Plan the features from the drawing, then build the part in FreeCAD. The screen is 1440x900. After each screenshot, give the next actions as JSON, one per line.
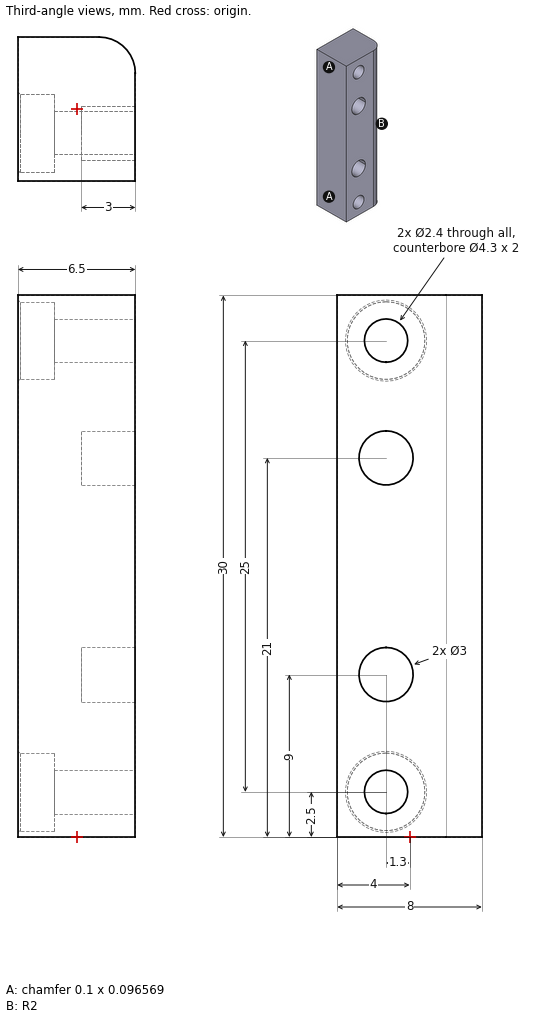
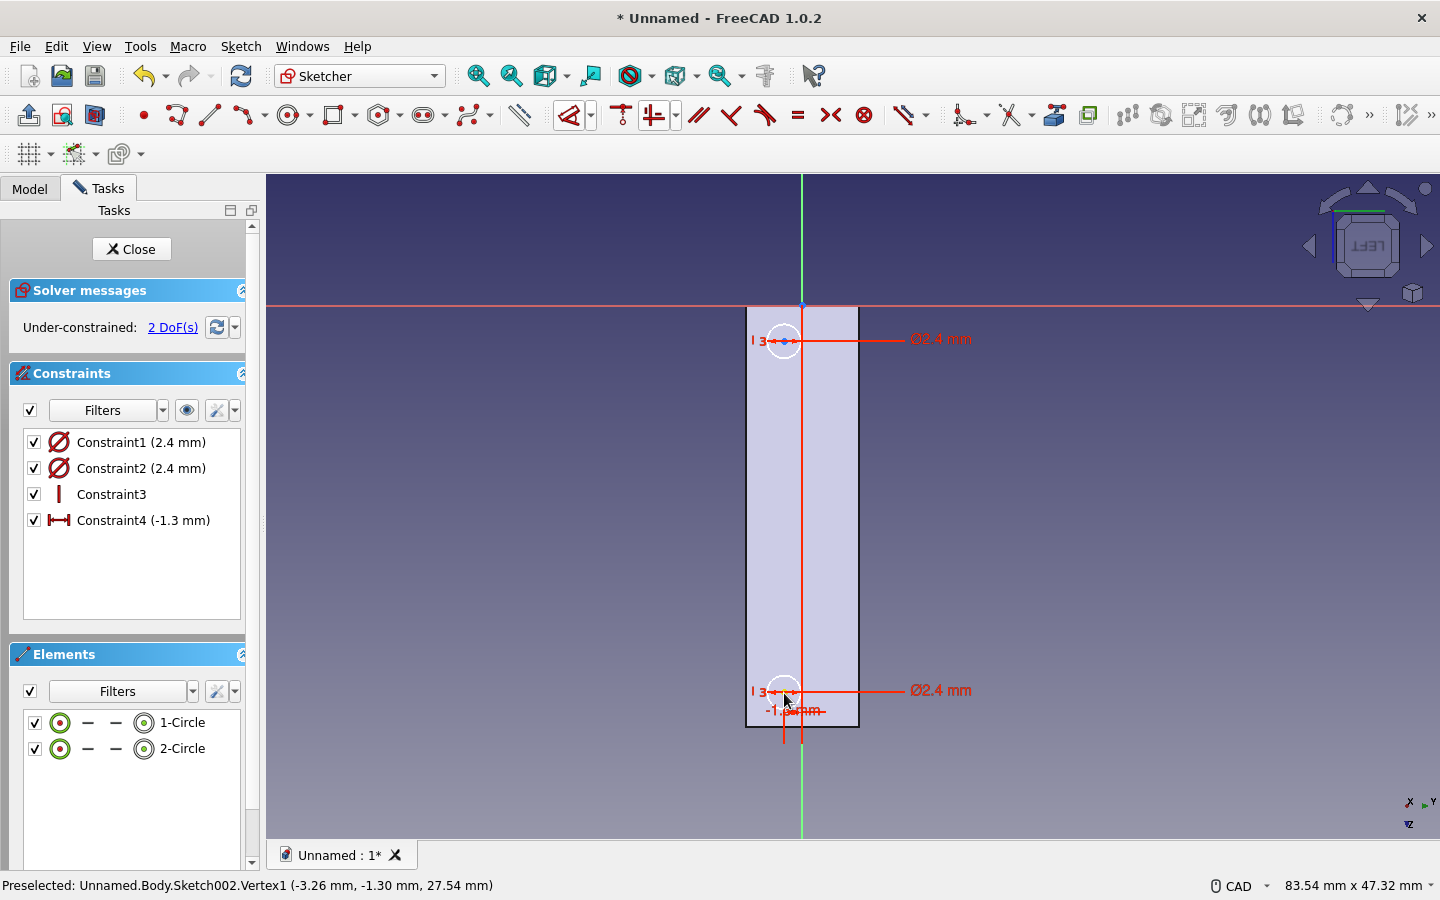
{"action": "left_click", "coordinate": [784, 341]}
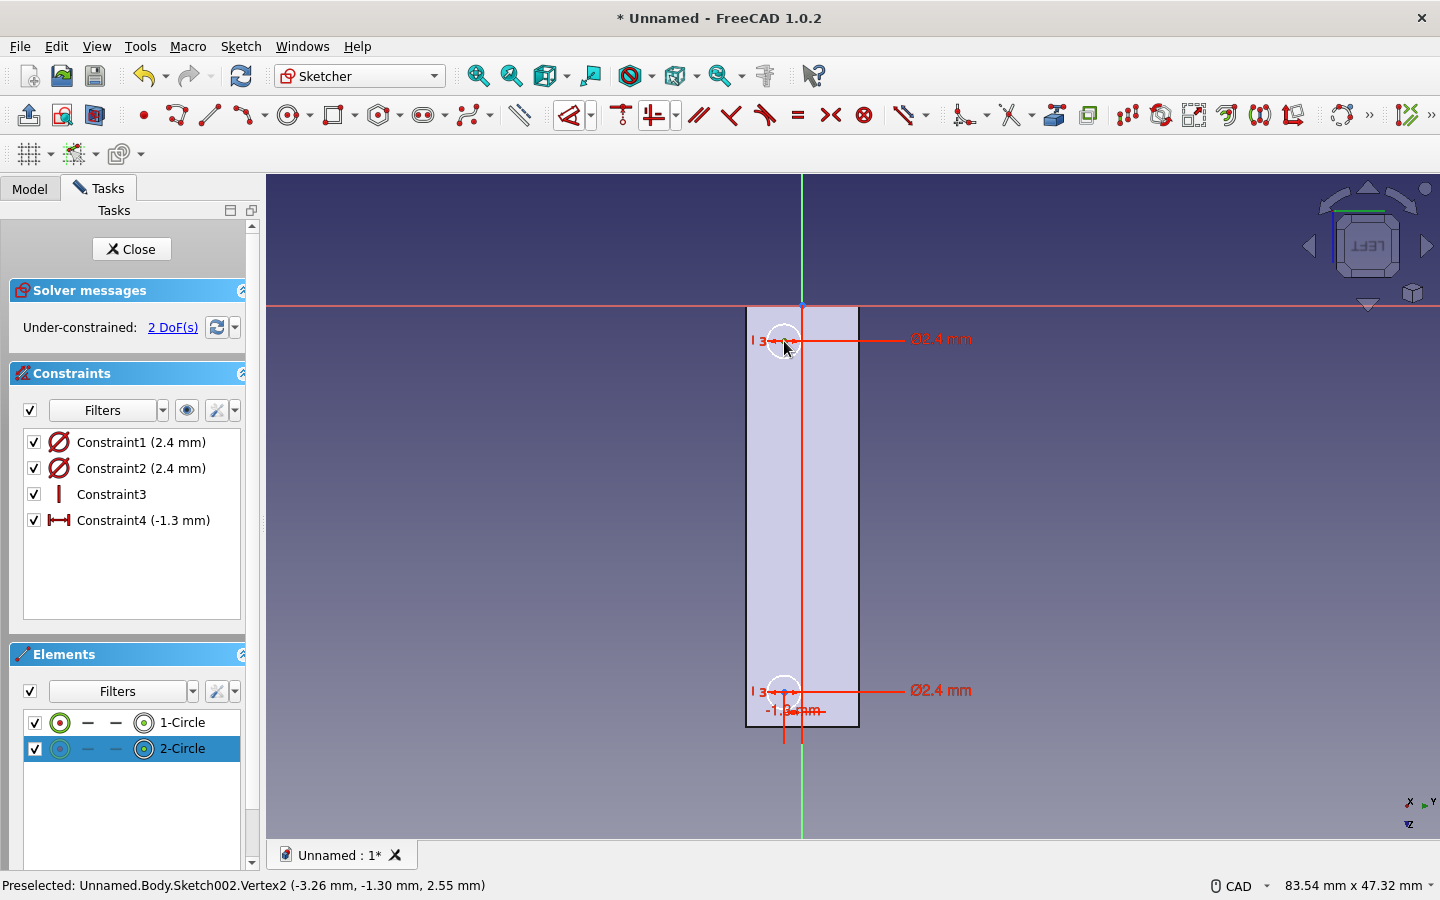
{"action": "left_click", "coordinate": [590, 116]}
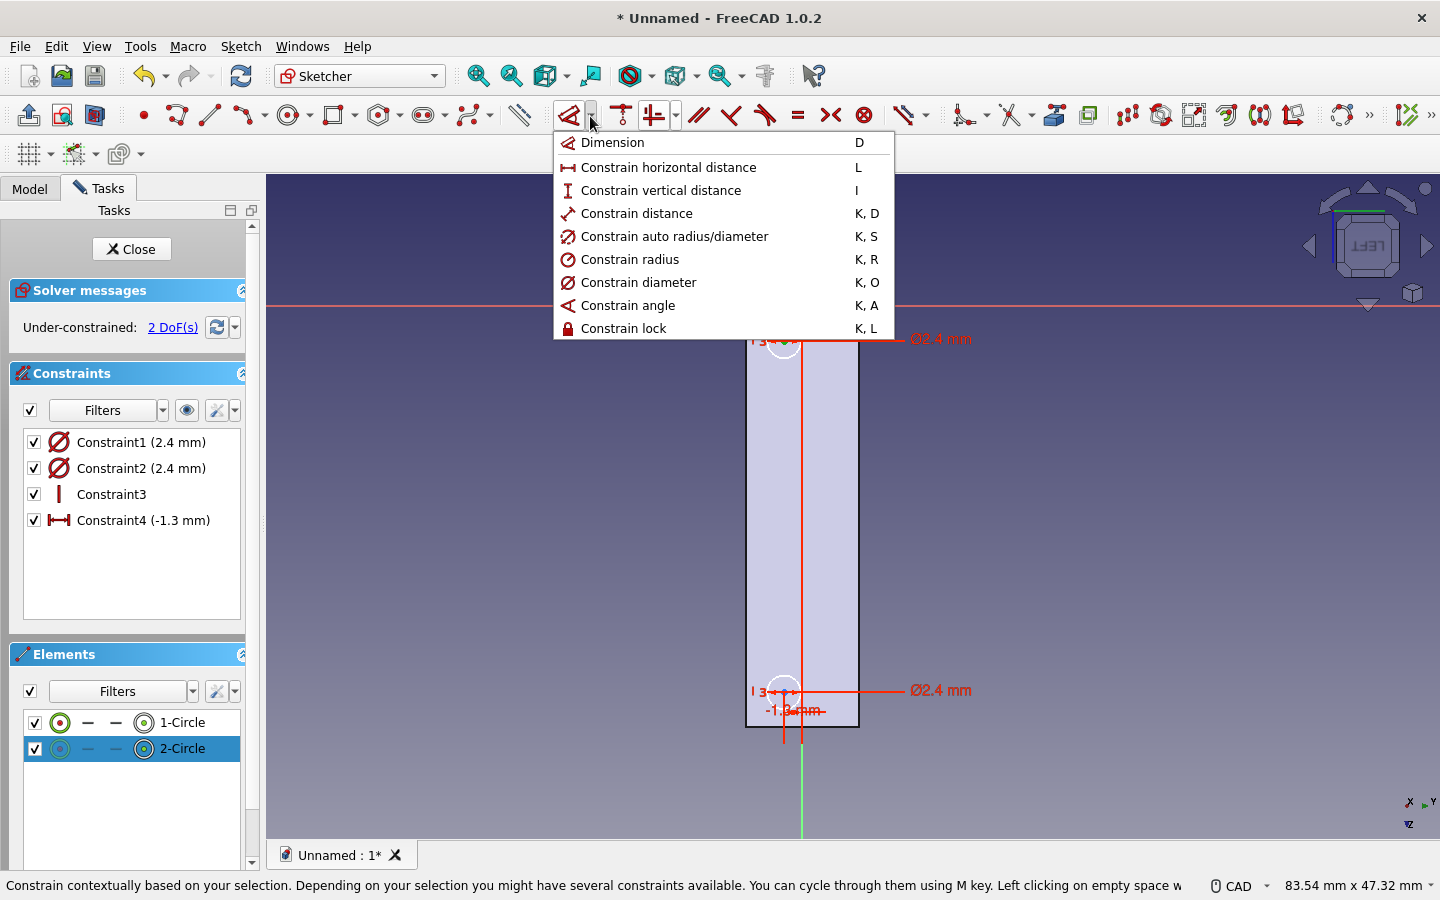
{"action": "left_click", "coordinate": [724, 190]}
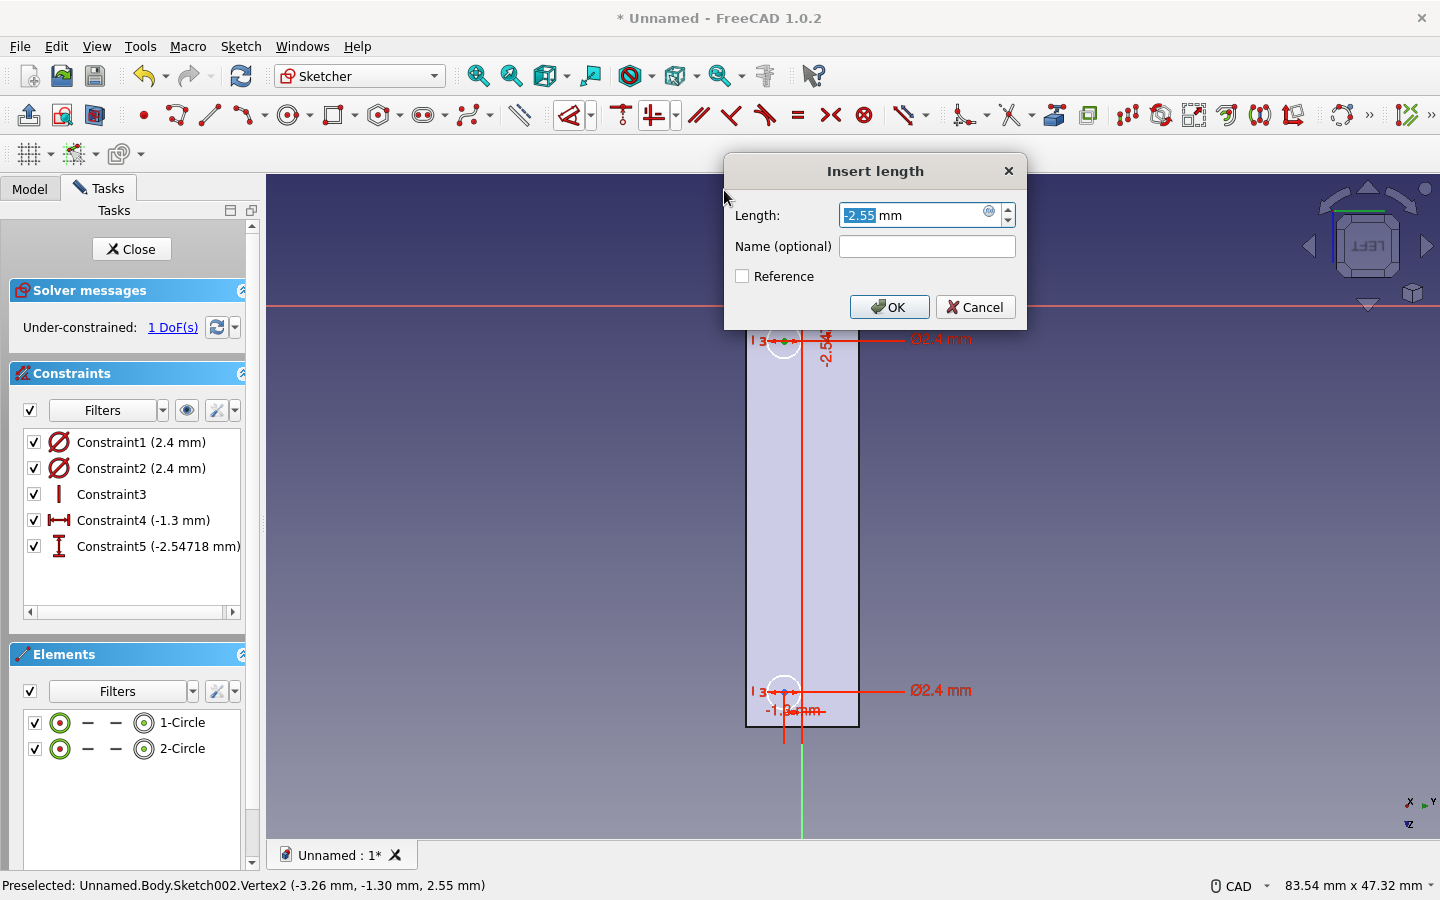
{"action": "type", "text": "-2.5"}
{"action": "key", "text": "Return"}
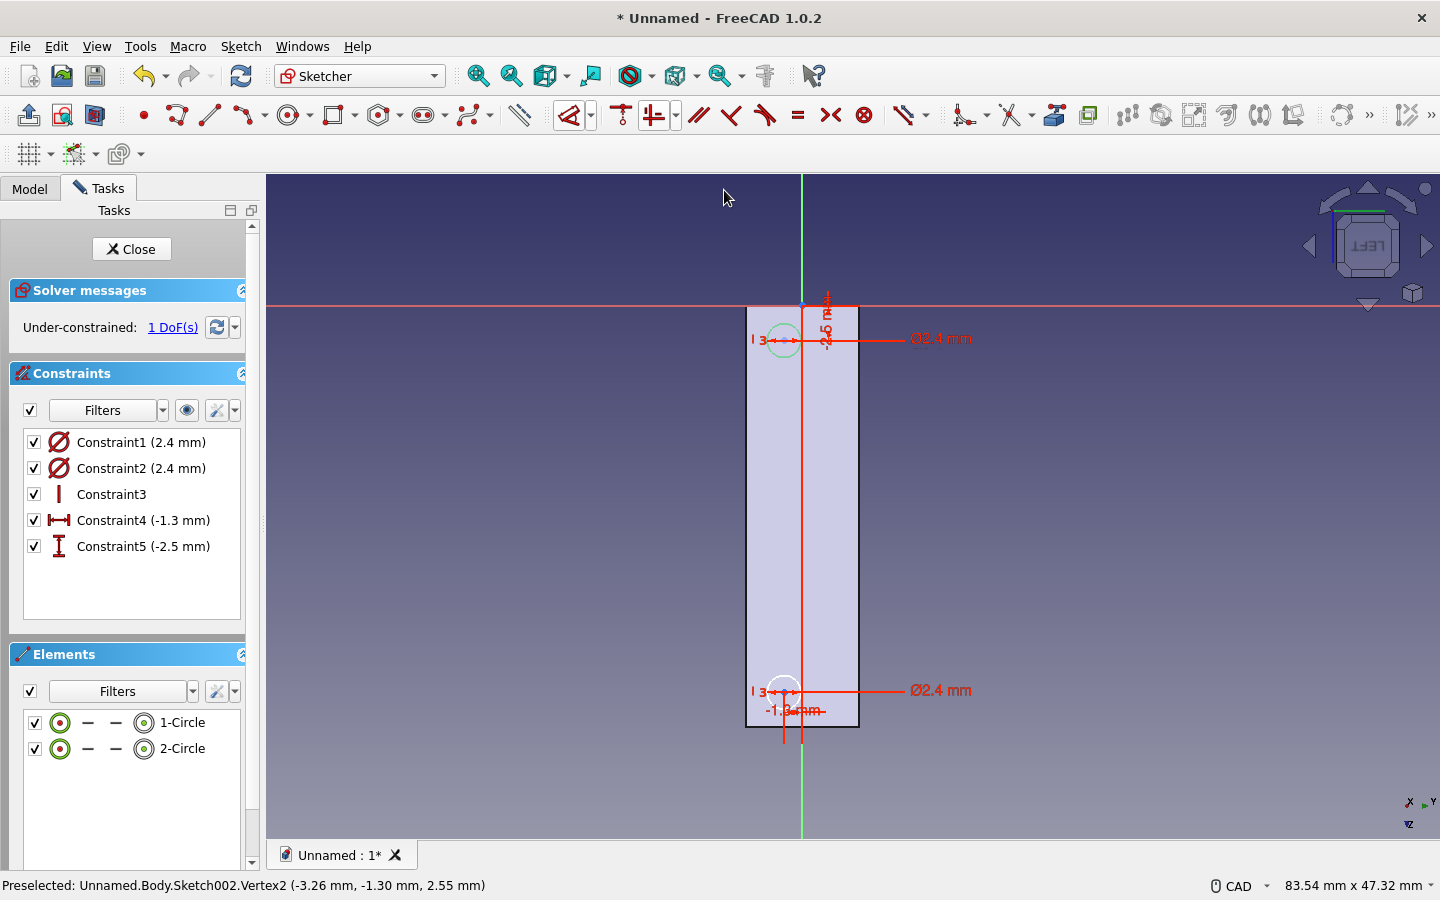
{"action": "left_click", "coordinate": [784, 692]}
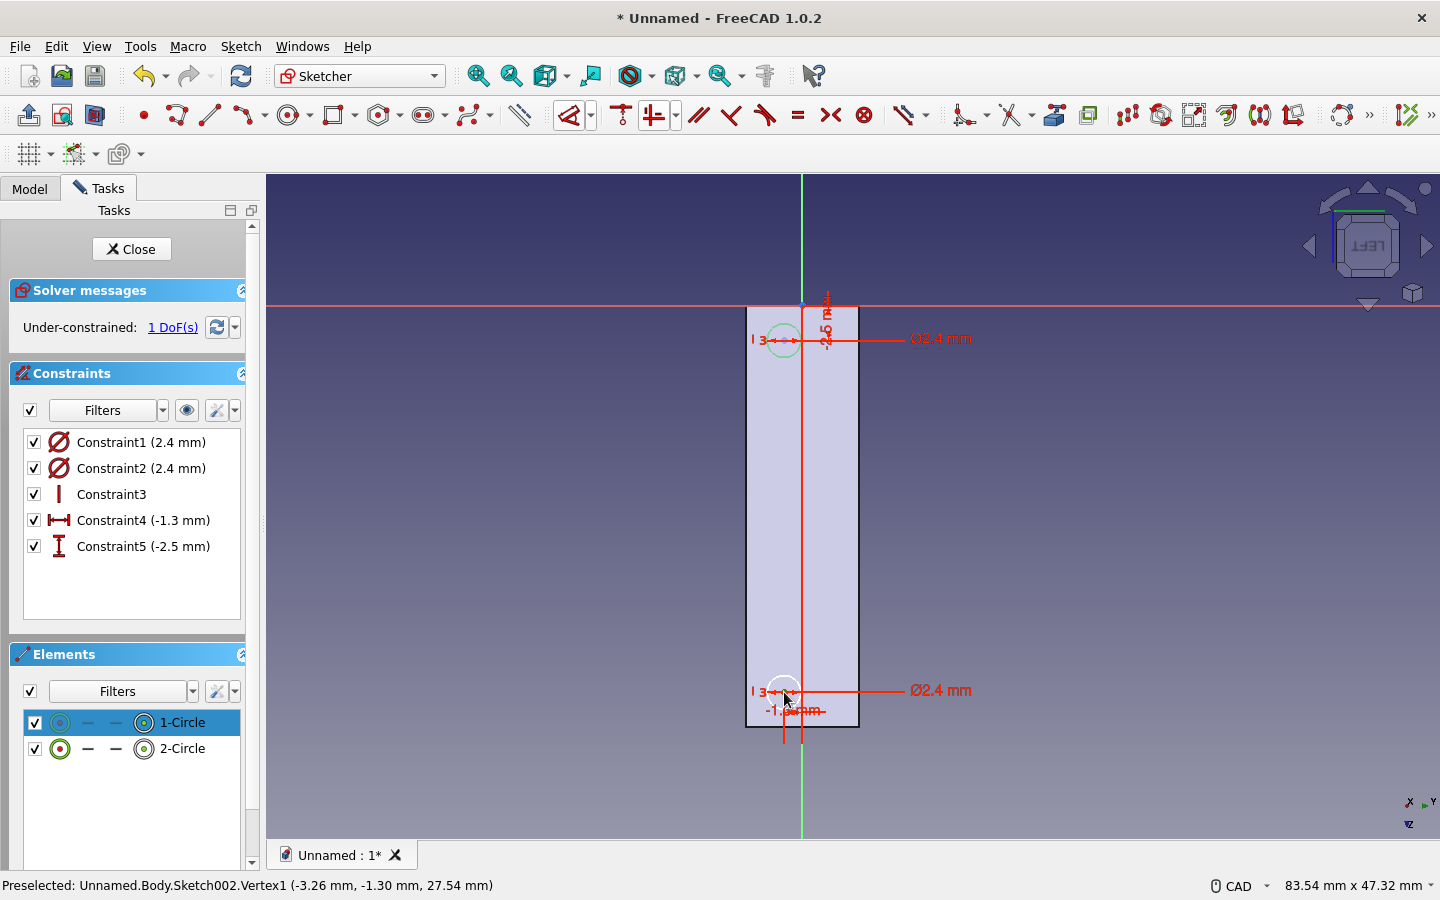
{"action": "left_click", "coordinate": [784, 341]}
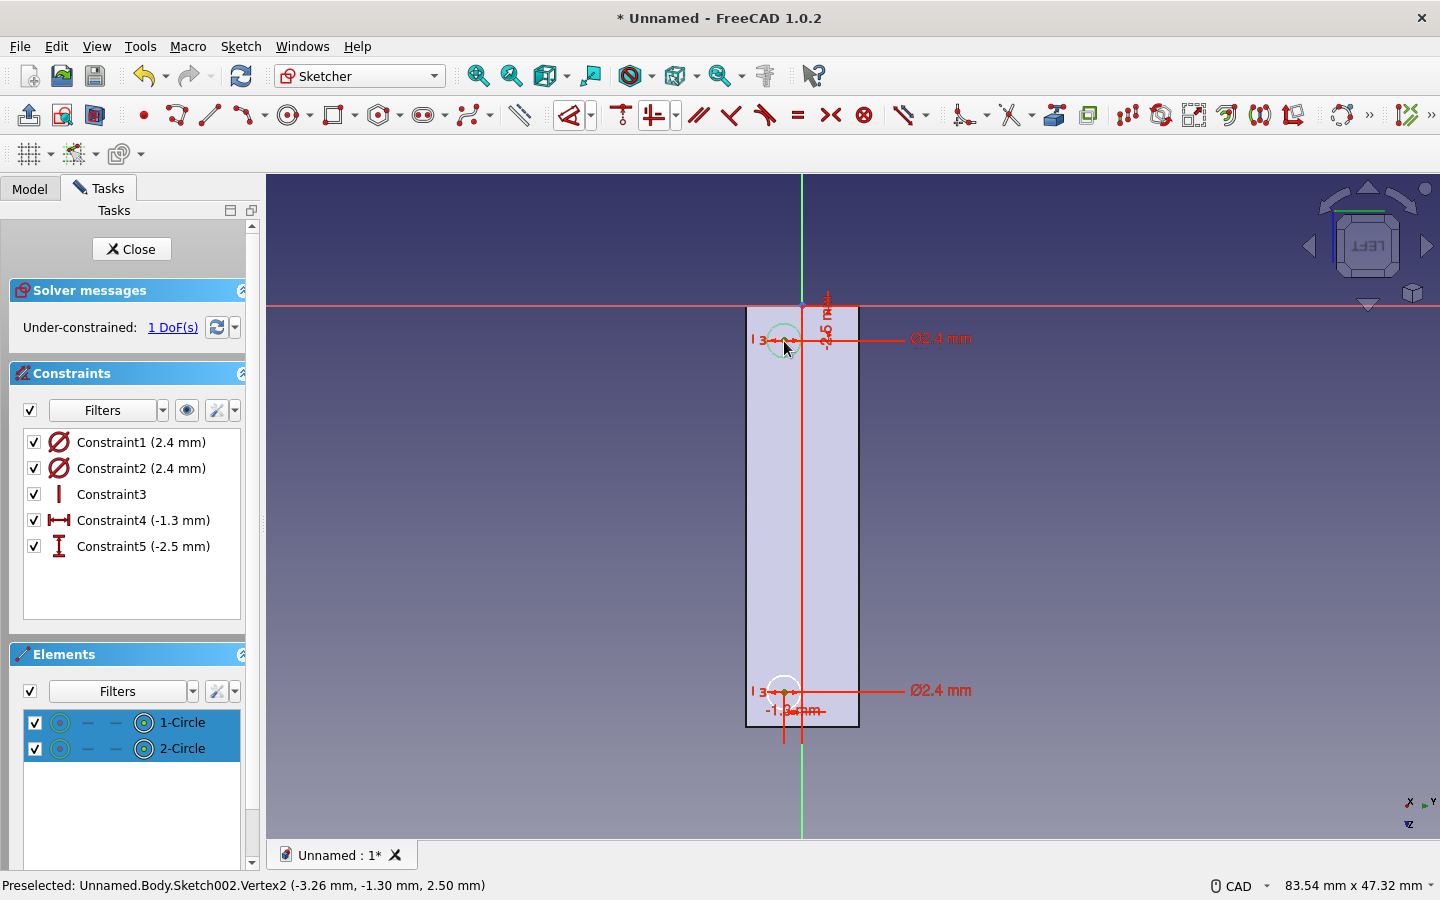
{"action": "left_click", "coordinate": [590, 116]}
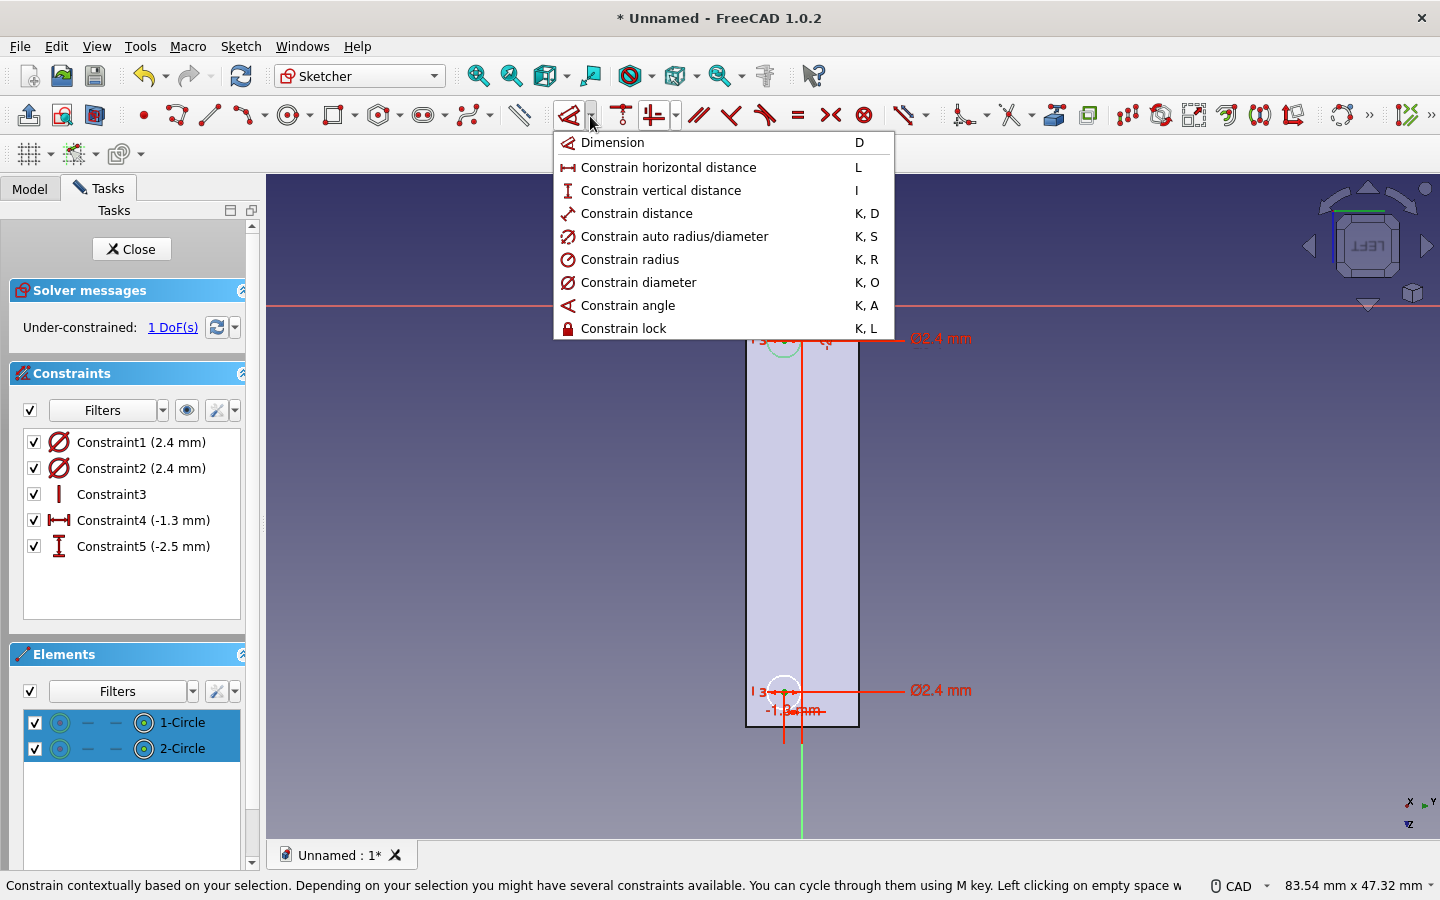
{"action": "left_click", "coordinate": [724, 190]}